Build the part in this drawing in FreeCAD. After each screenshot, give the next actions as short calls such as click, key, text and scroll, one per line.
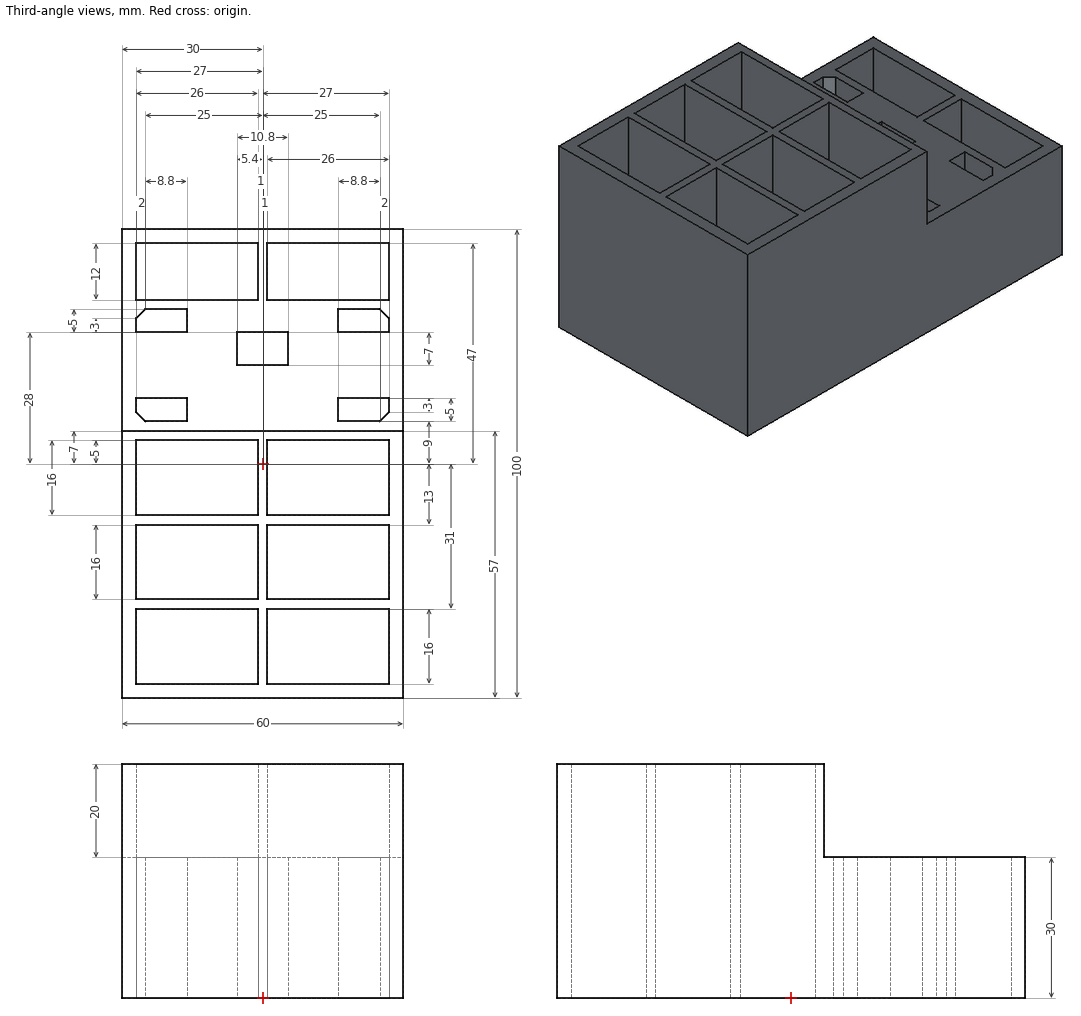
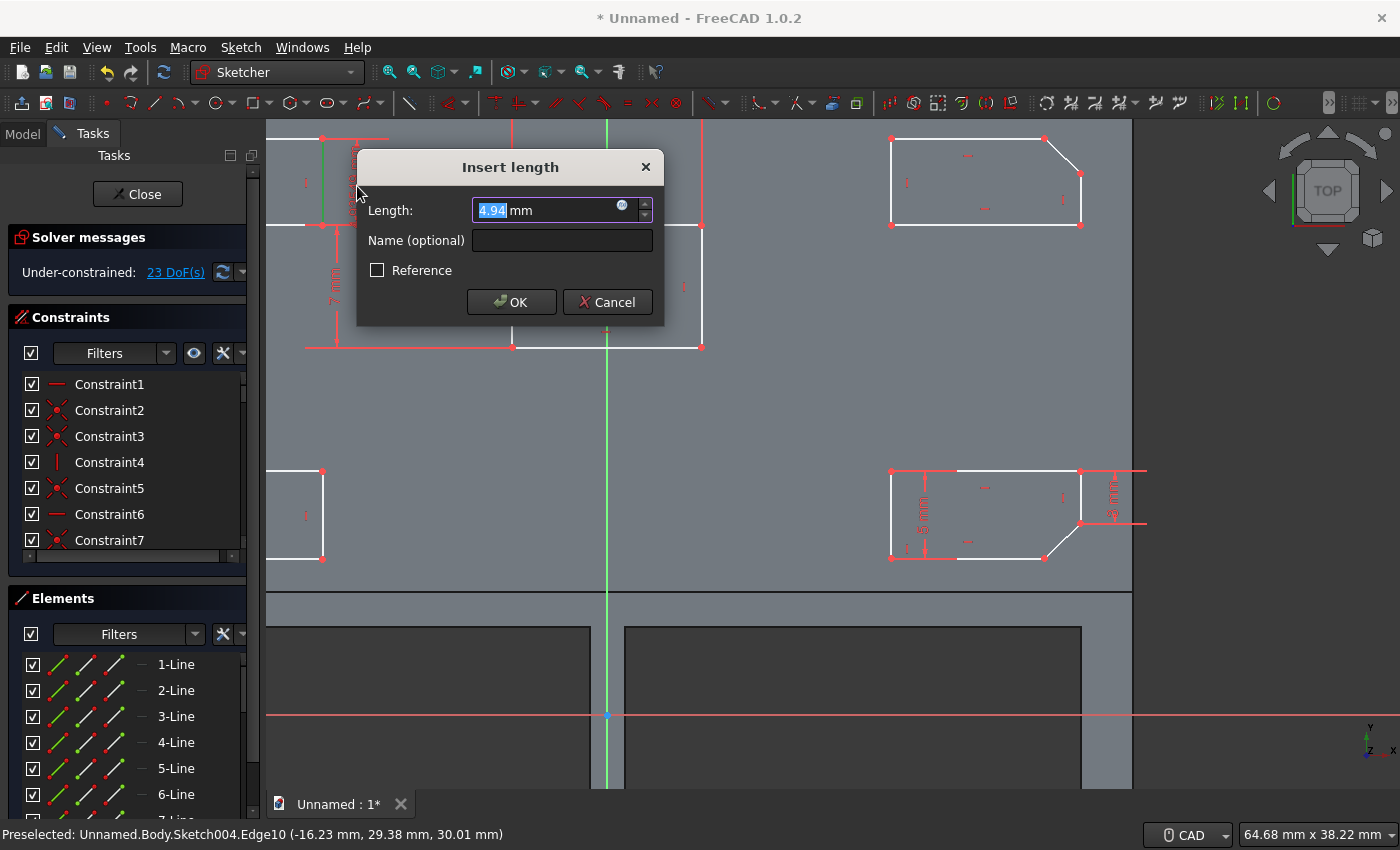
text(5)
key(Return)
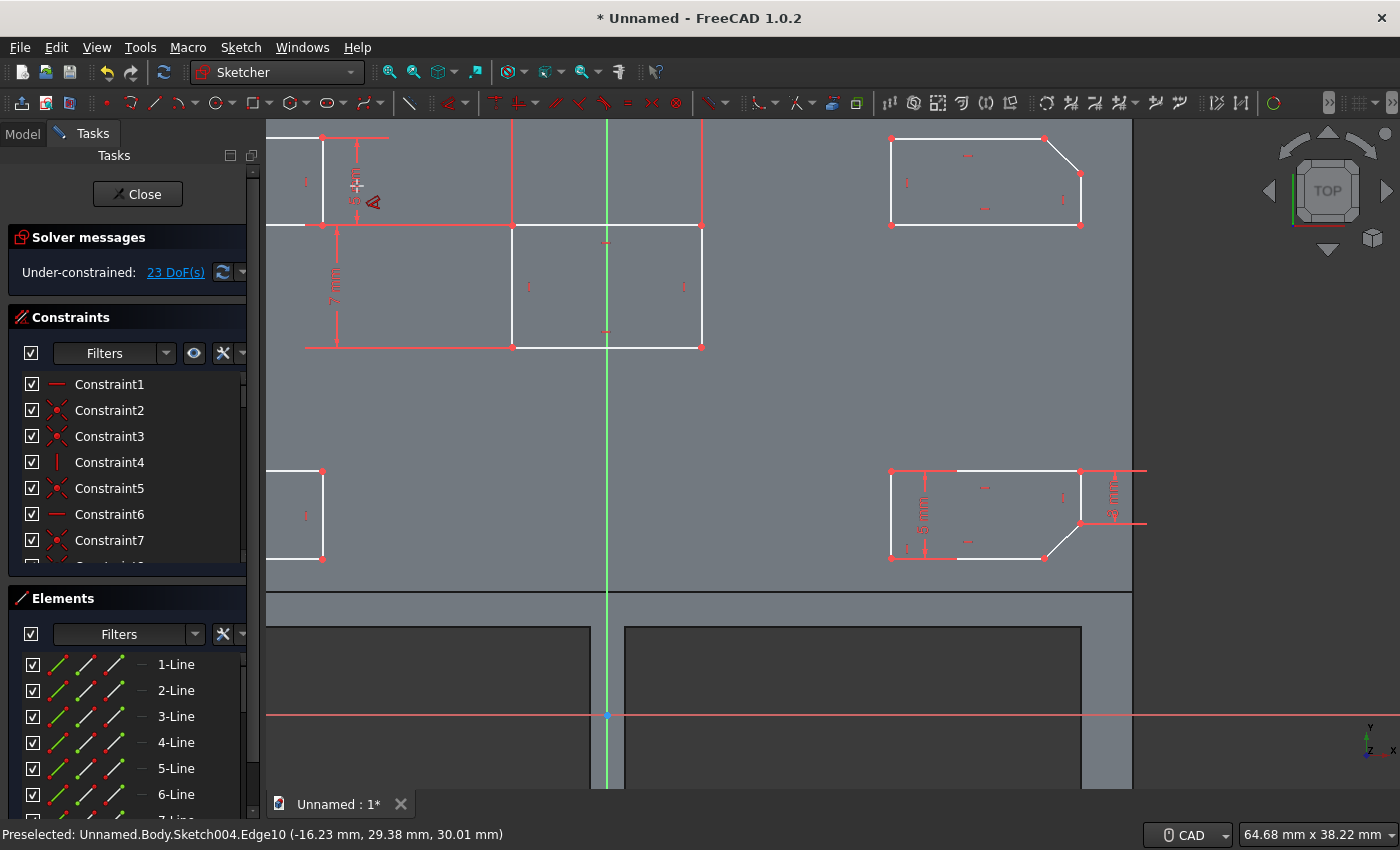
scroll(1084, 511, down, 2)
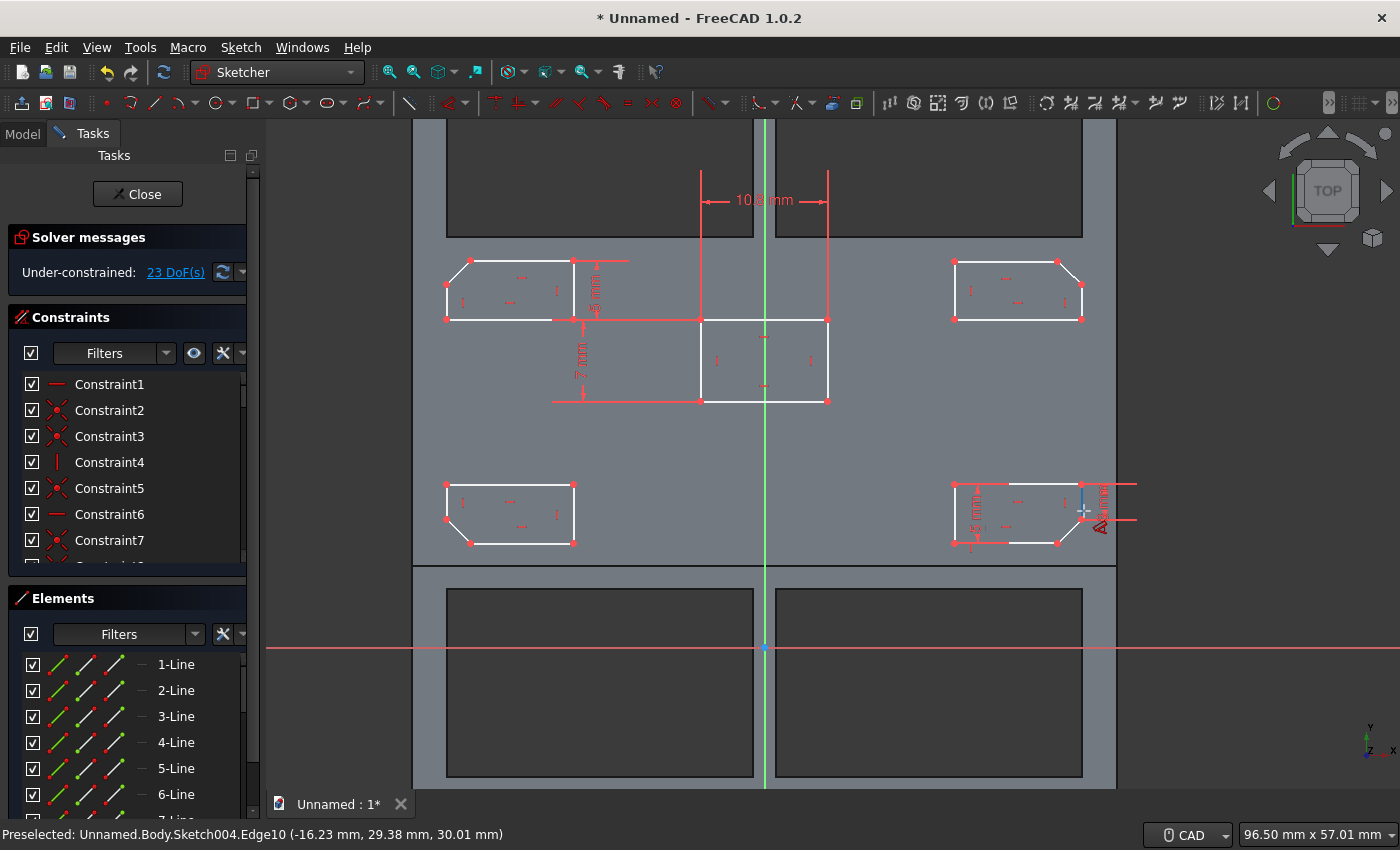
scroll(447, 295, up, 2)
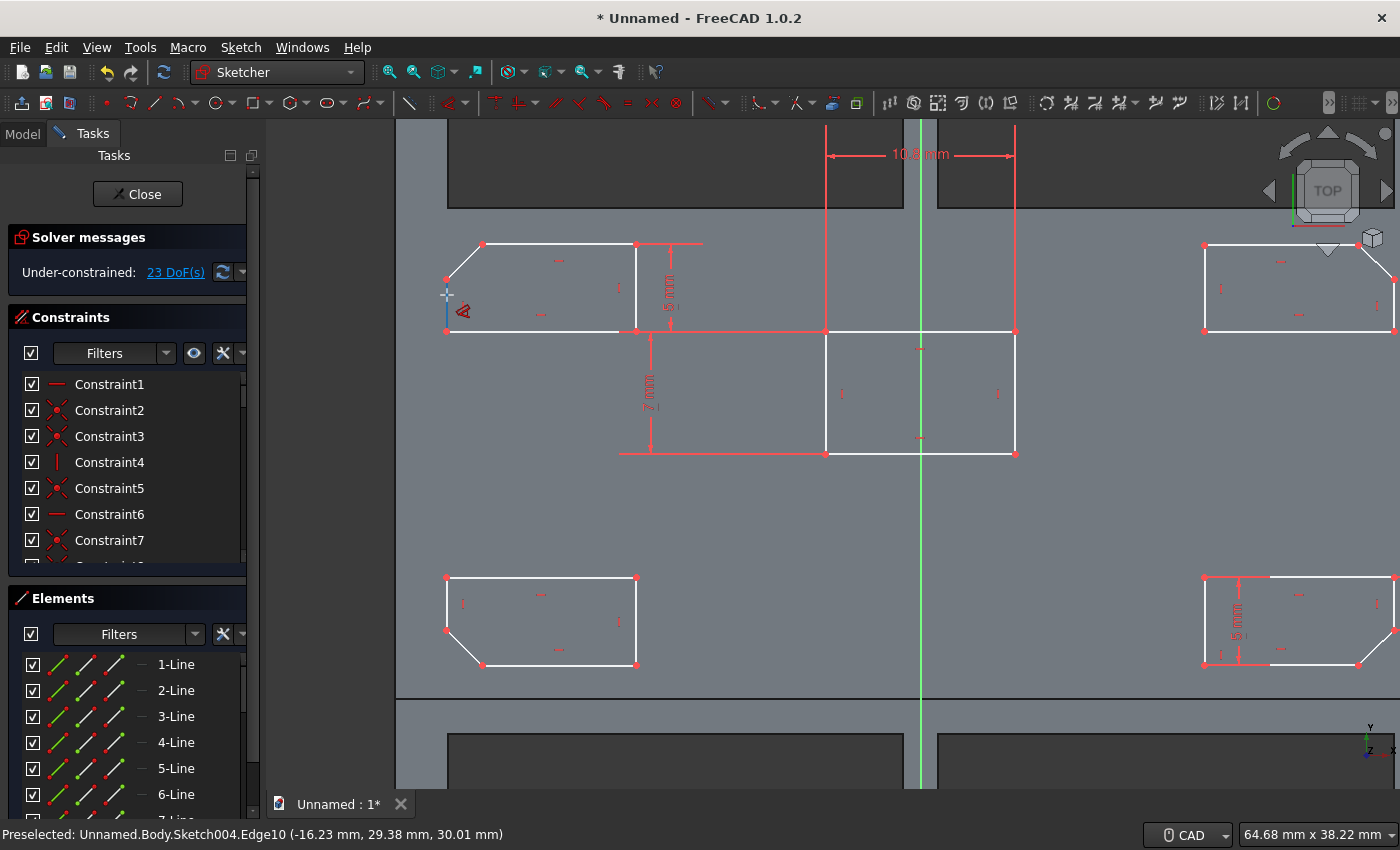
click(447, 295)
click(413, 306)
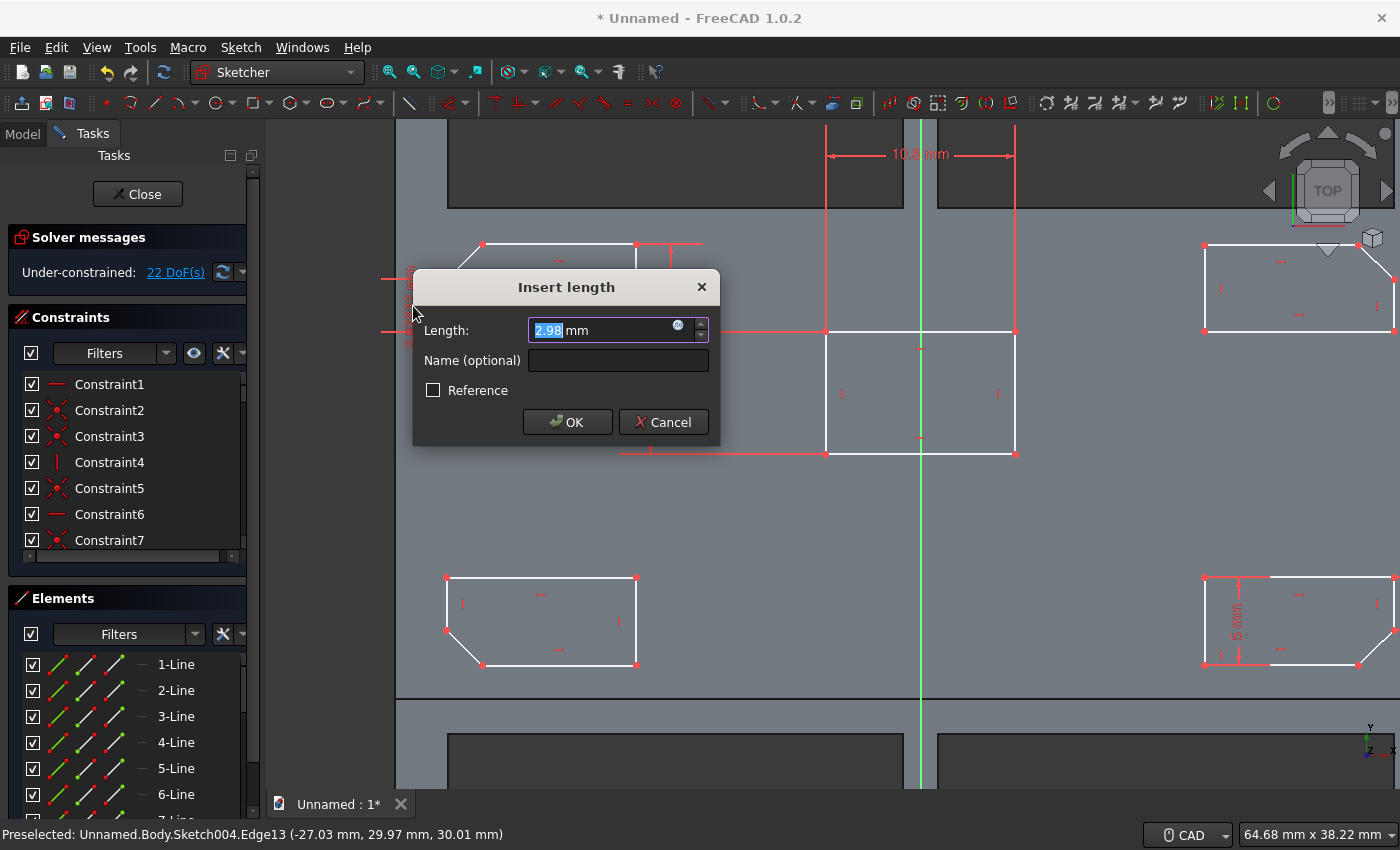
text(3)
key(Return)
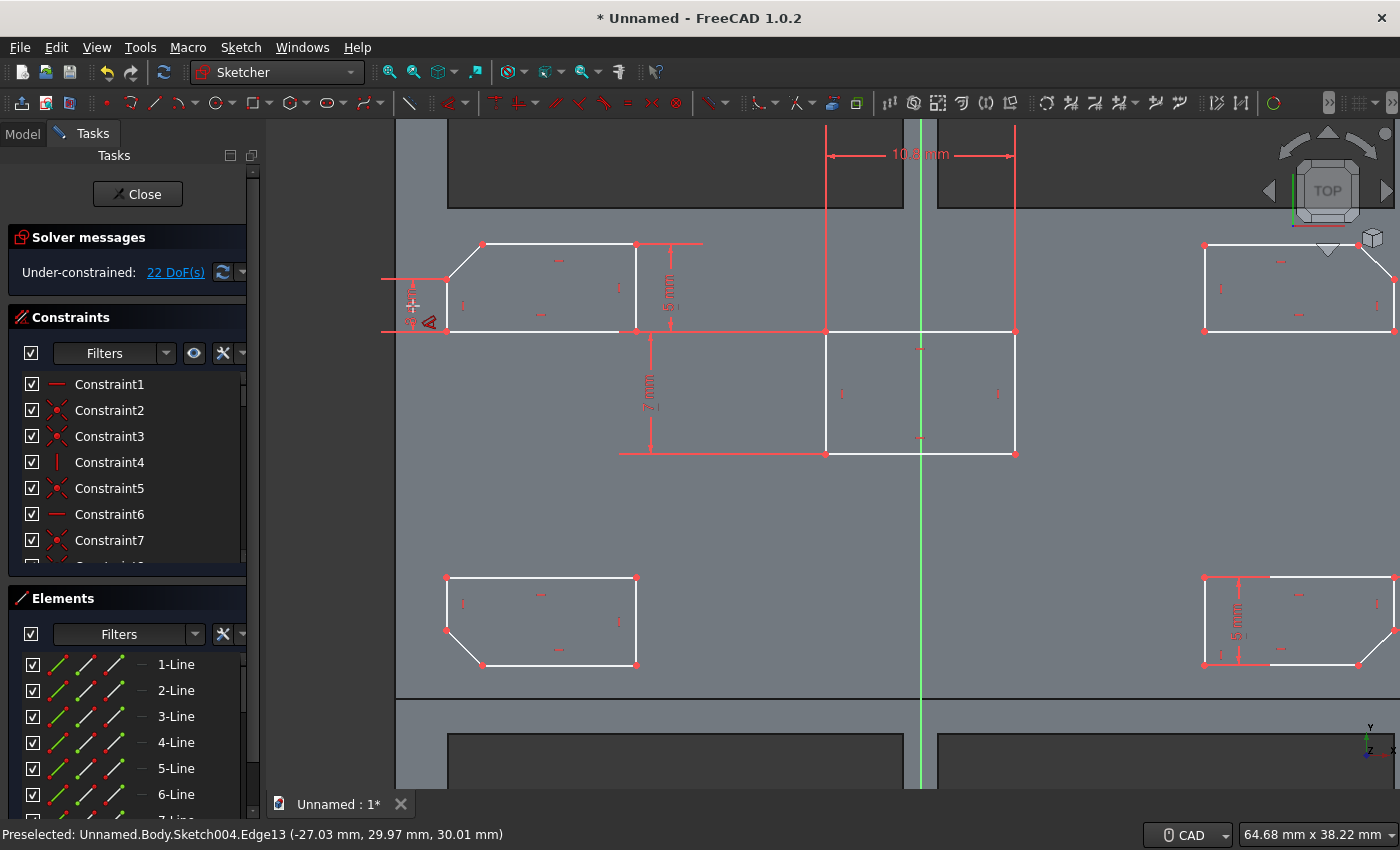
scroll(447, 295, down, 2)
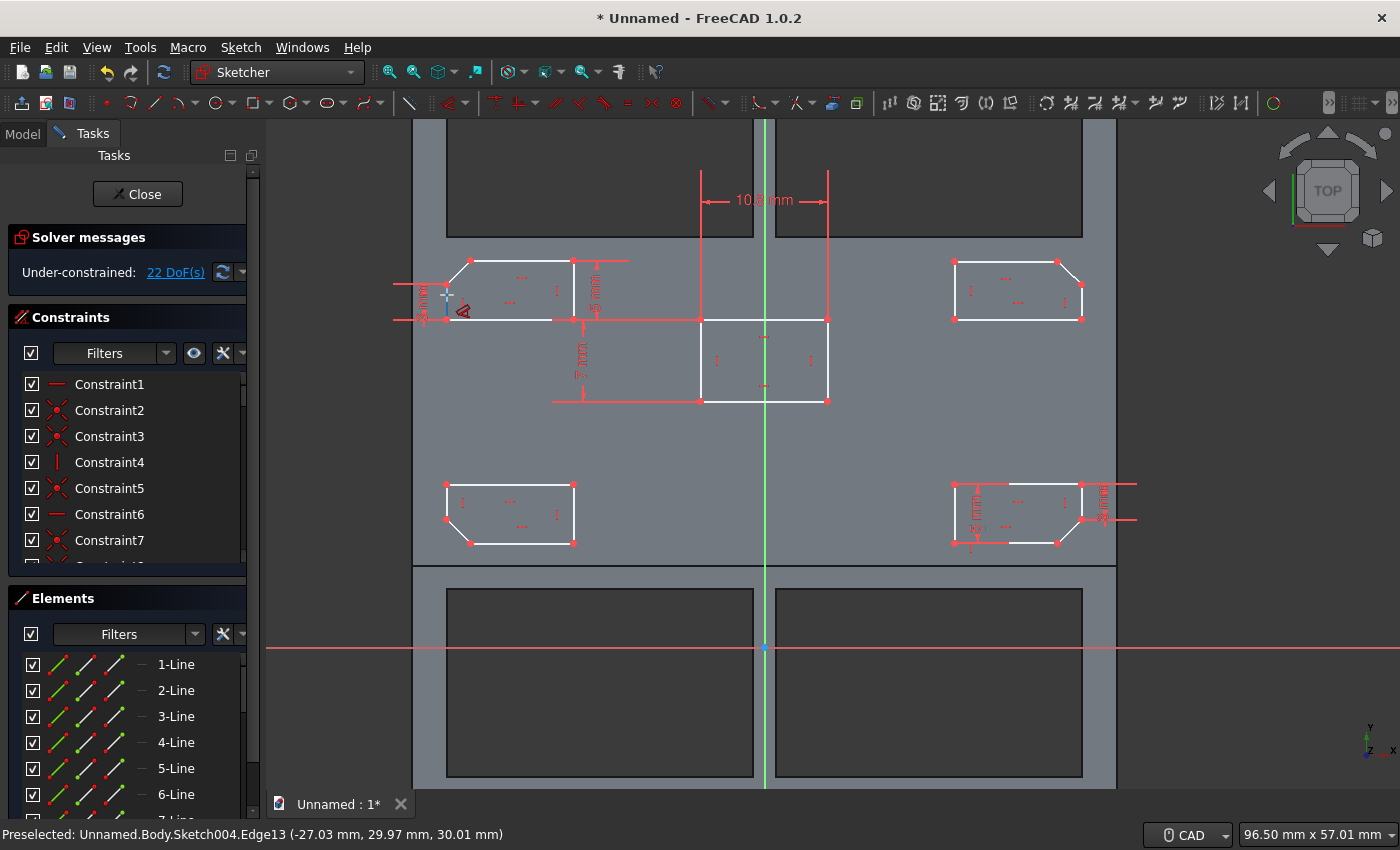
scroll(1082, 309, up, 2)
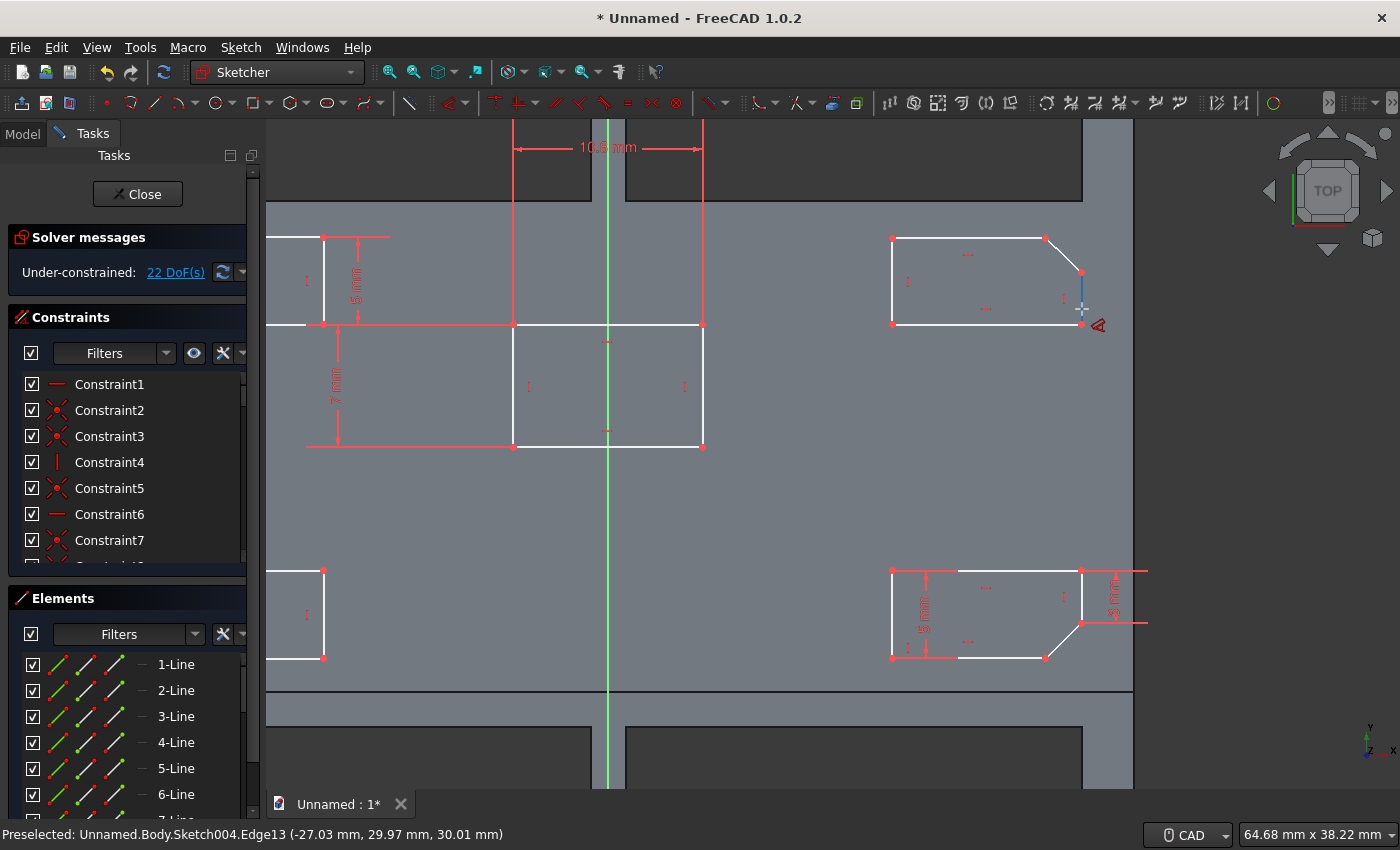
click(1082, 309)
click(1116, 299)